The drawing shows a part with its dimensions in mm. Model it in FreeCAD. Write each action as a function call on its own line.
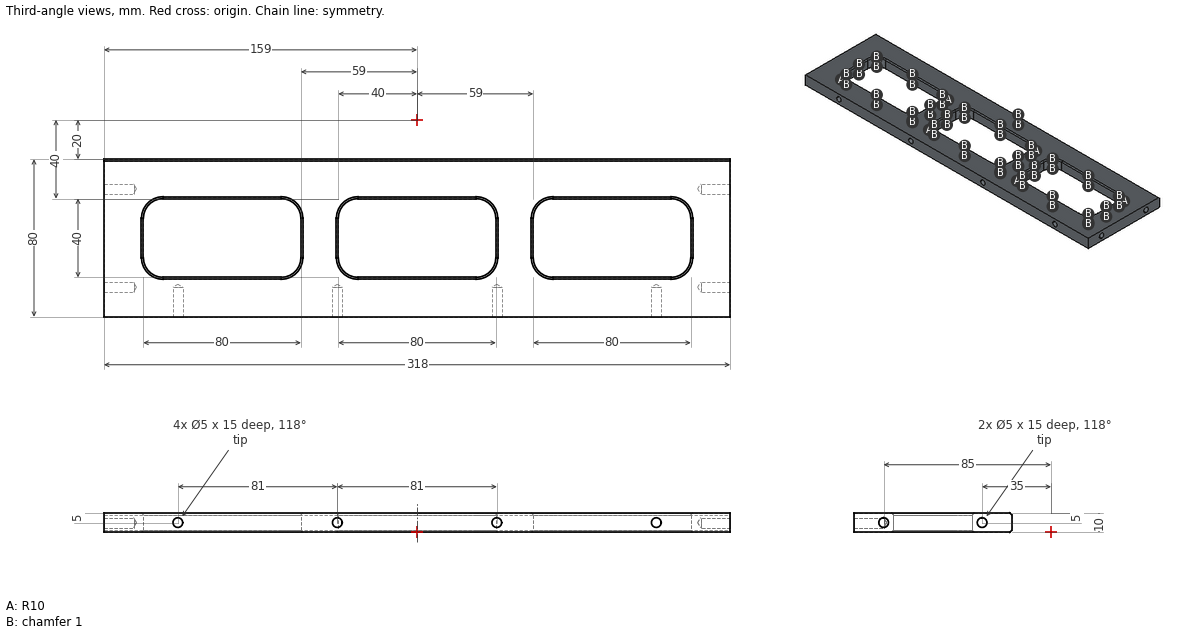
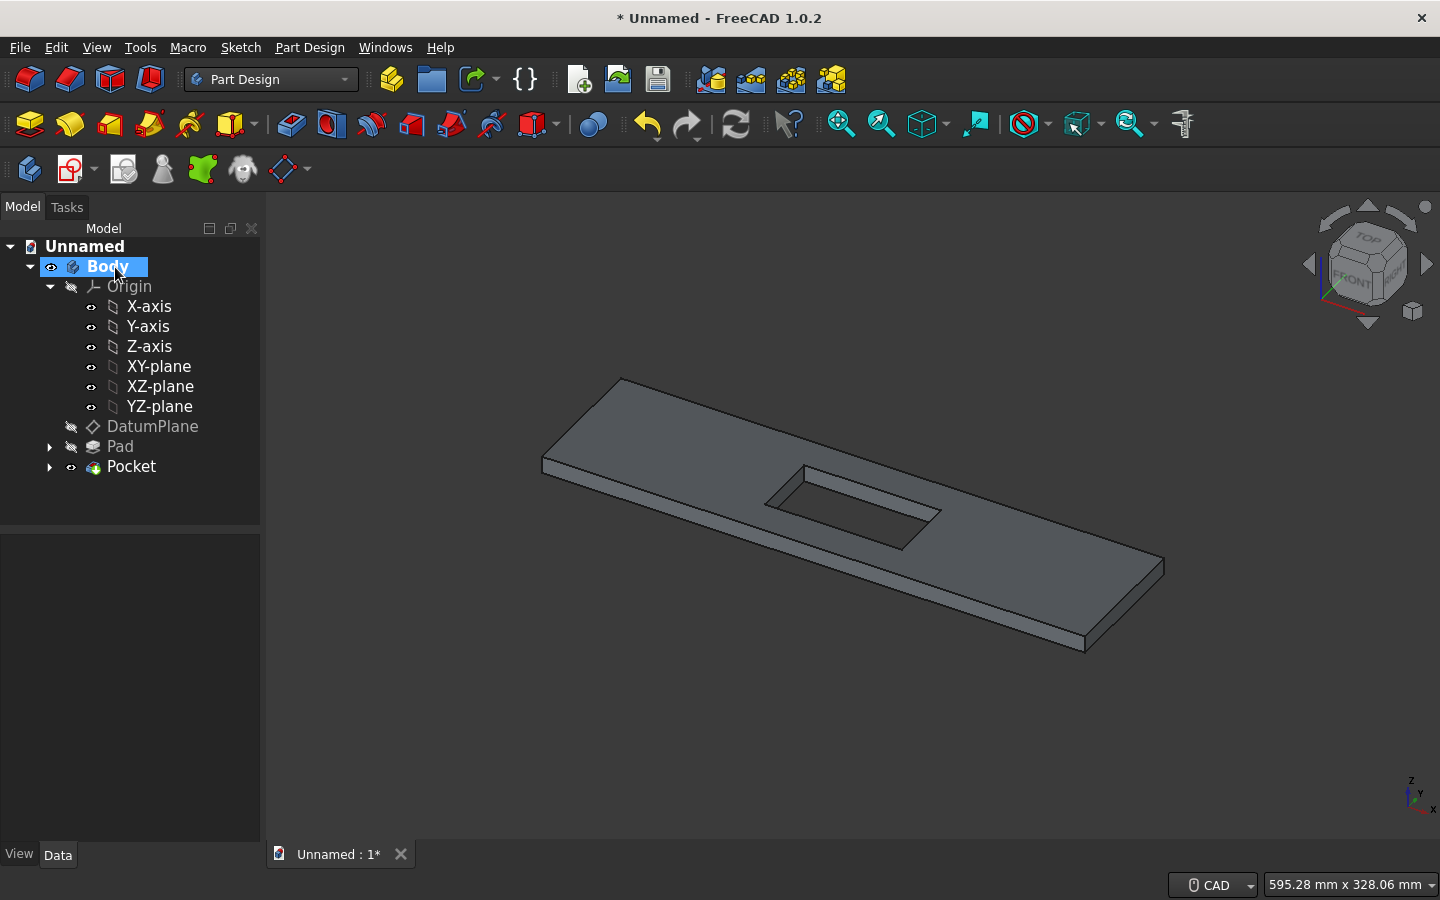
click(1008, 558)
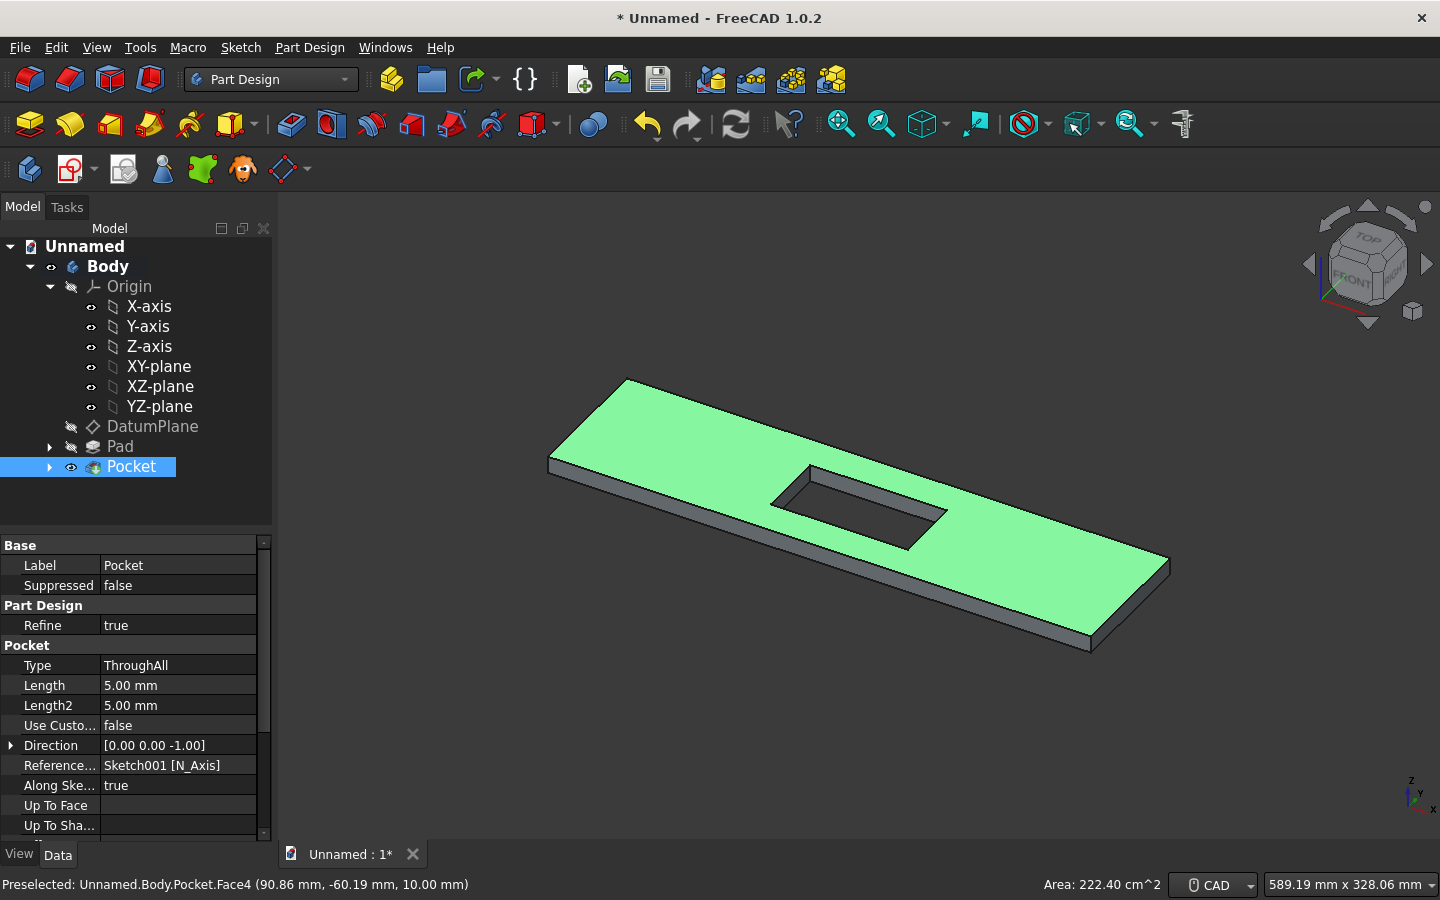
click(70, 170)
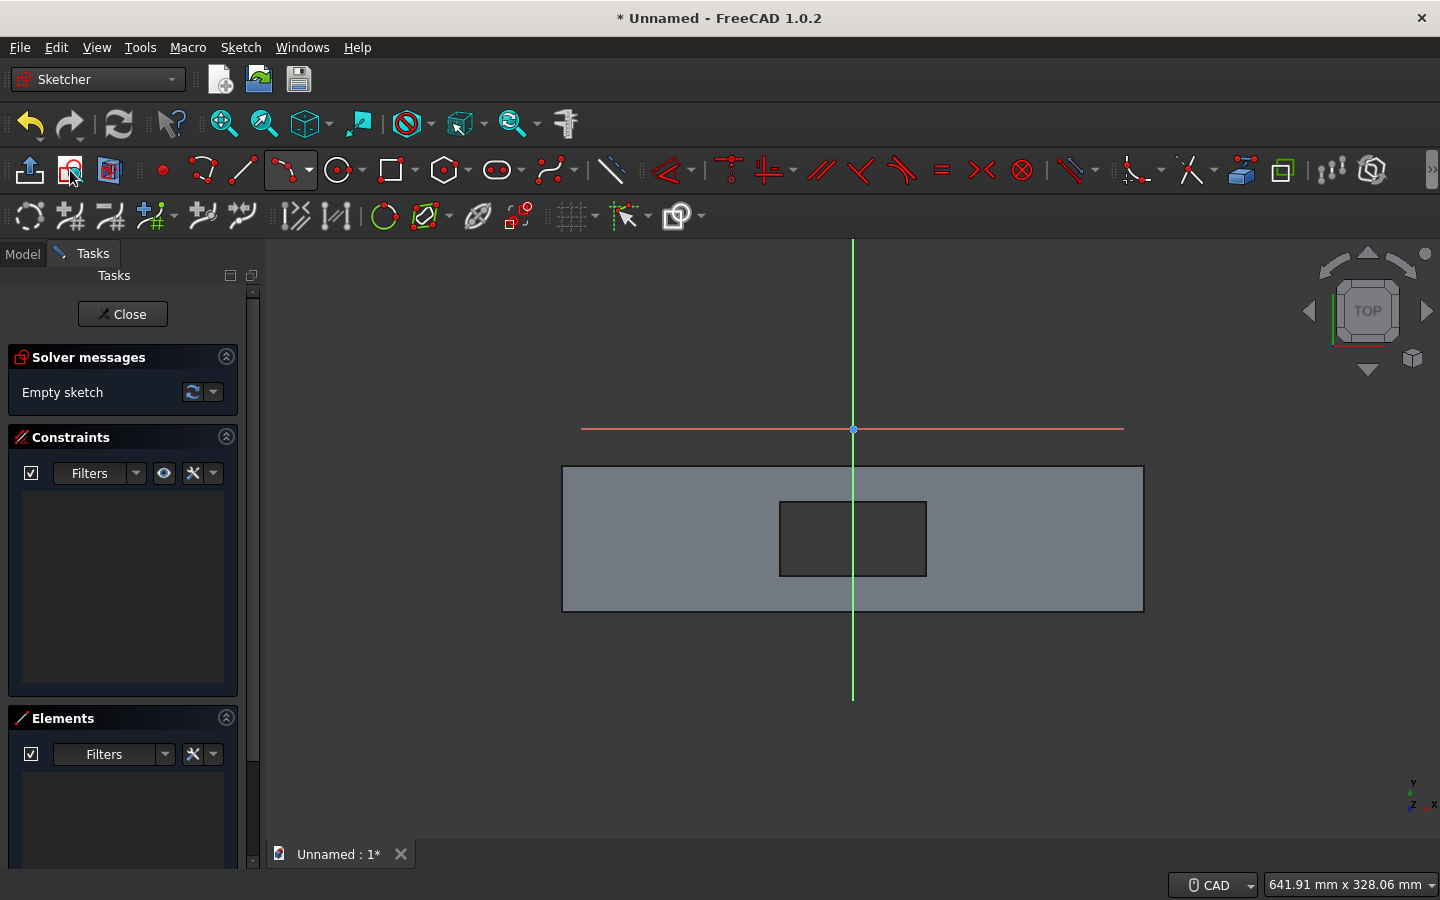
scroll(1094, 481, up, 5)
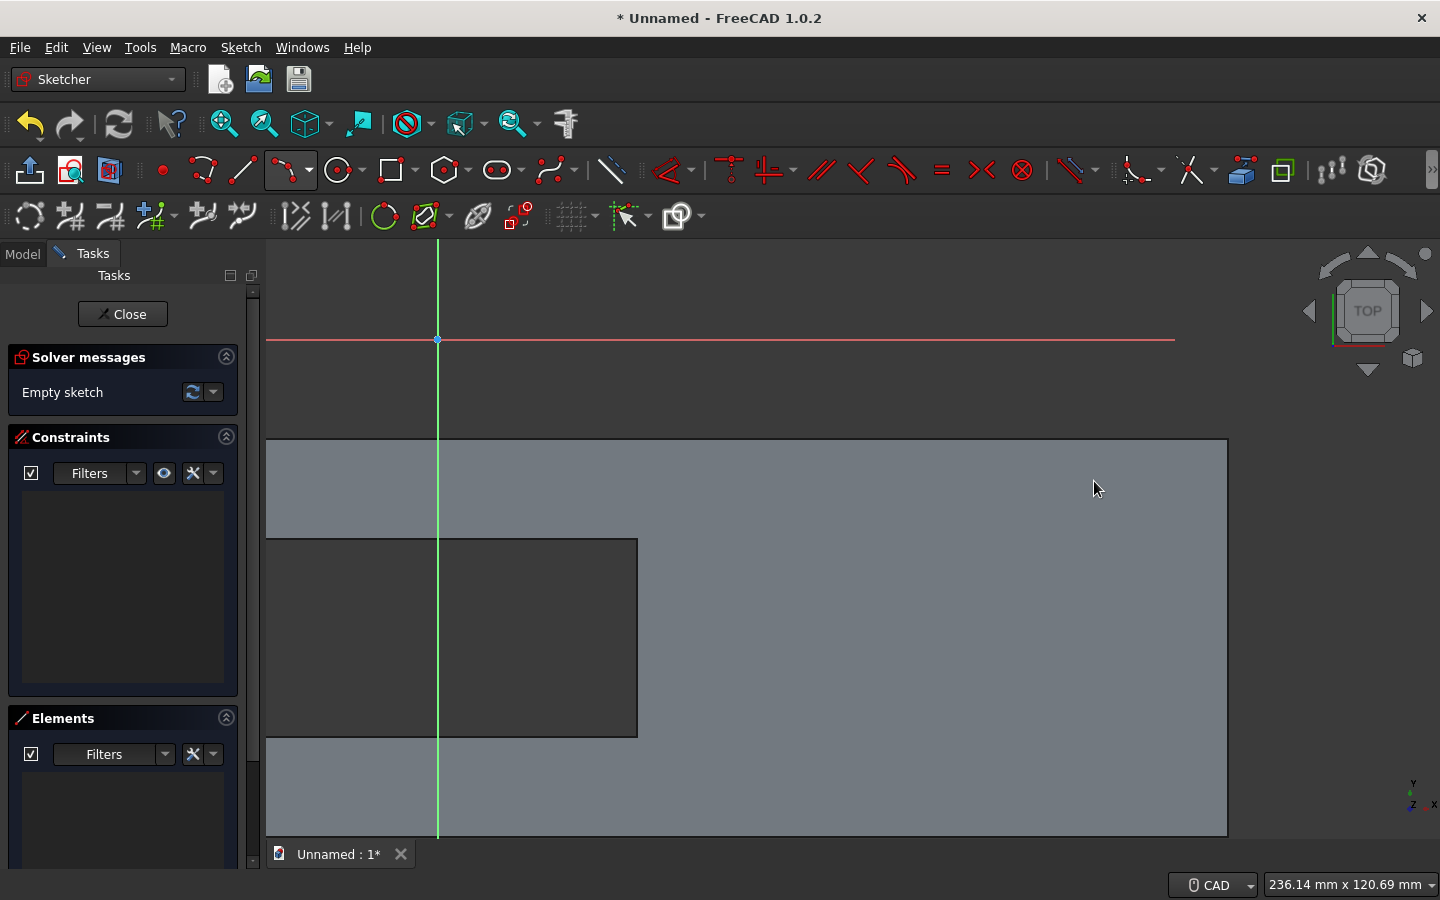
click(392, 170)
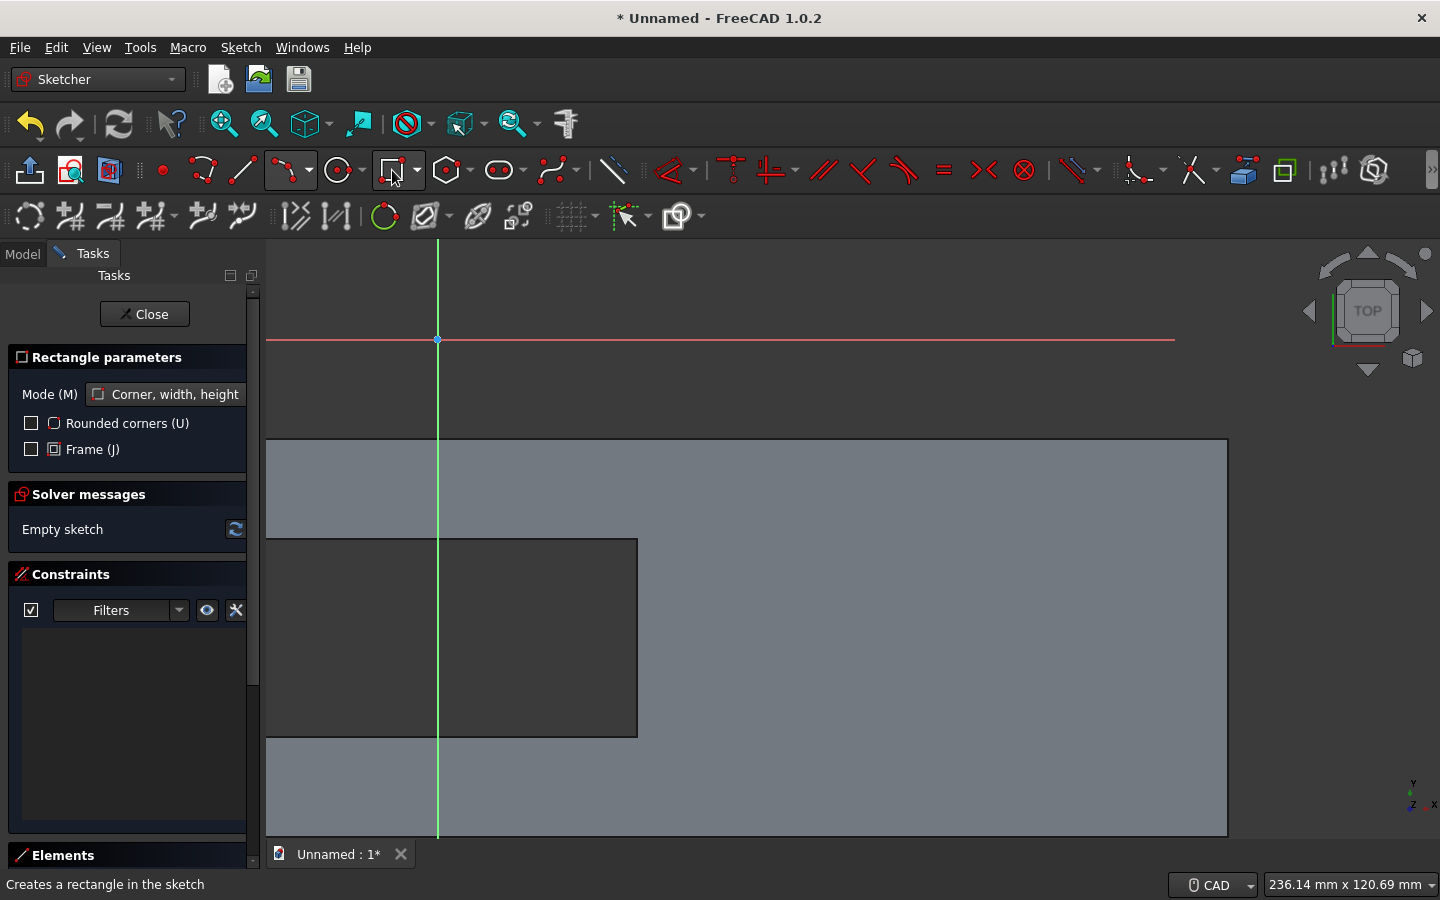
click(731, 539)
click(1129, 737)
key(Escape)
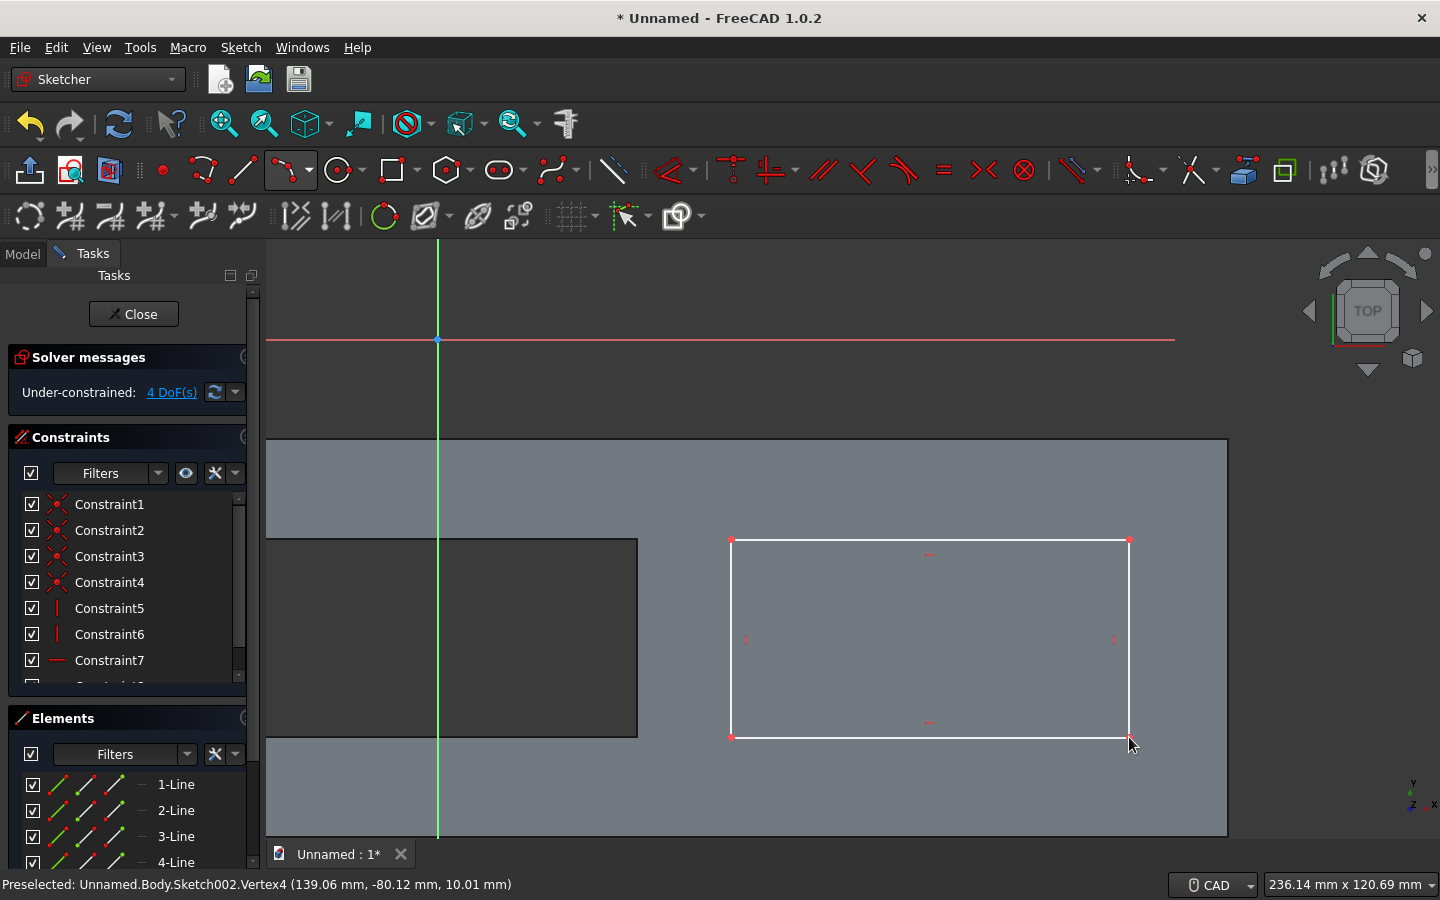
click(668, 170)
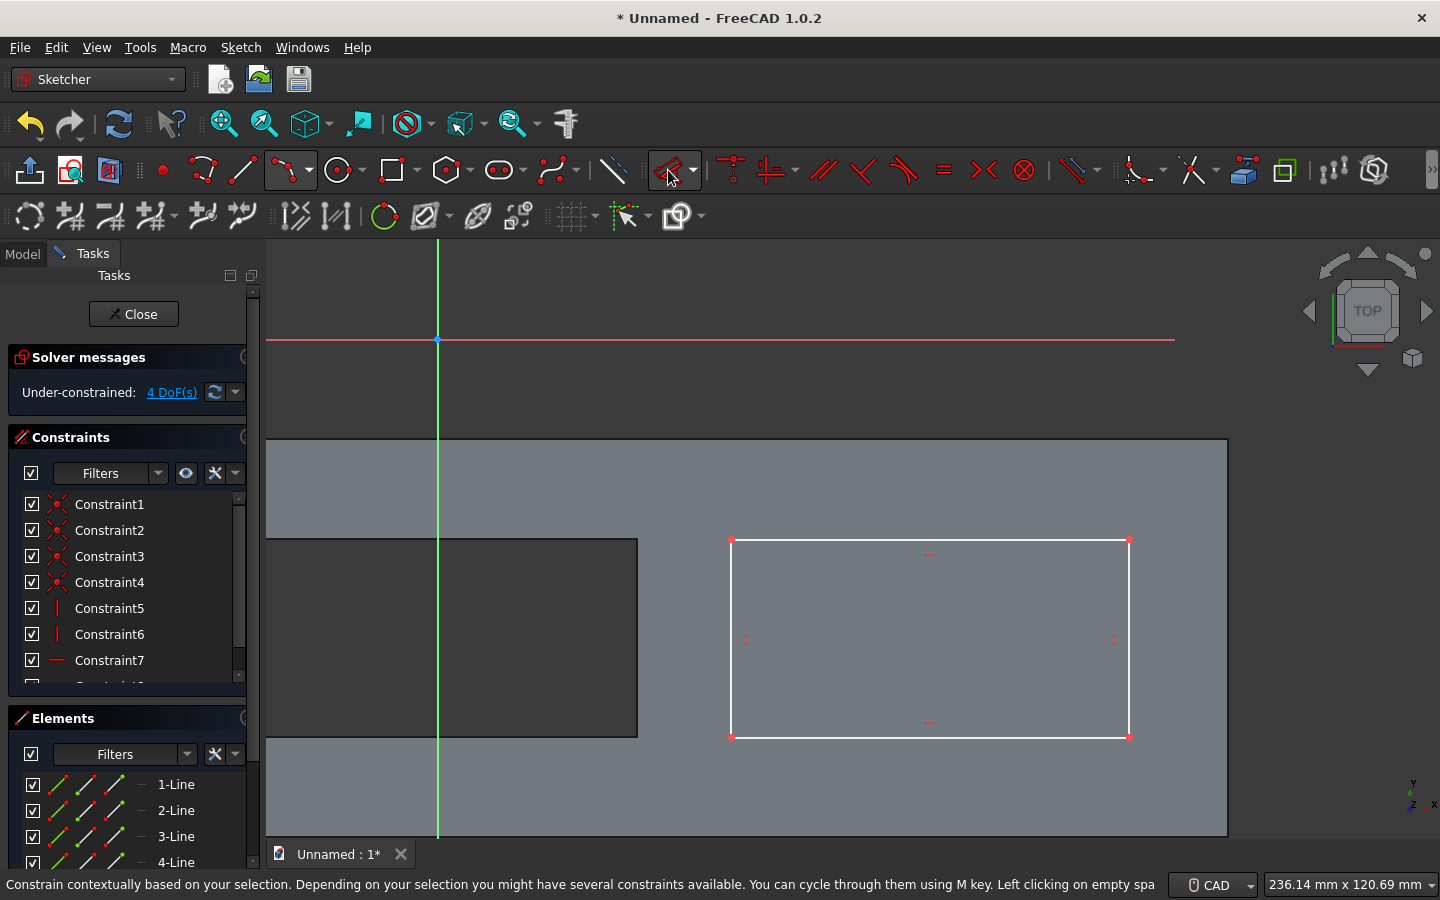
click(731, 599)
click(697, 639)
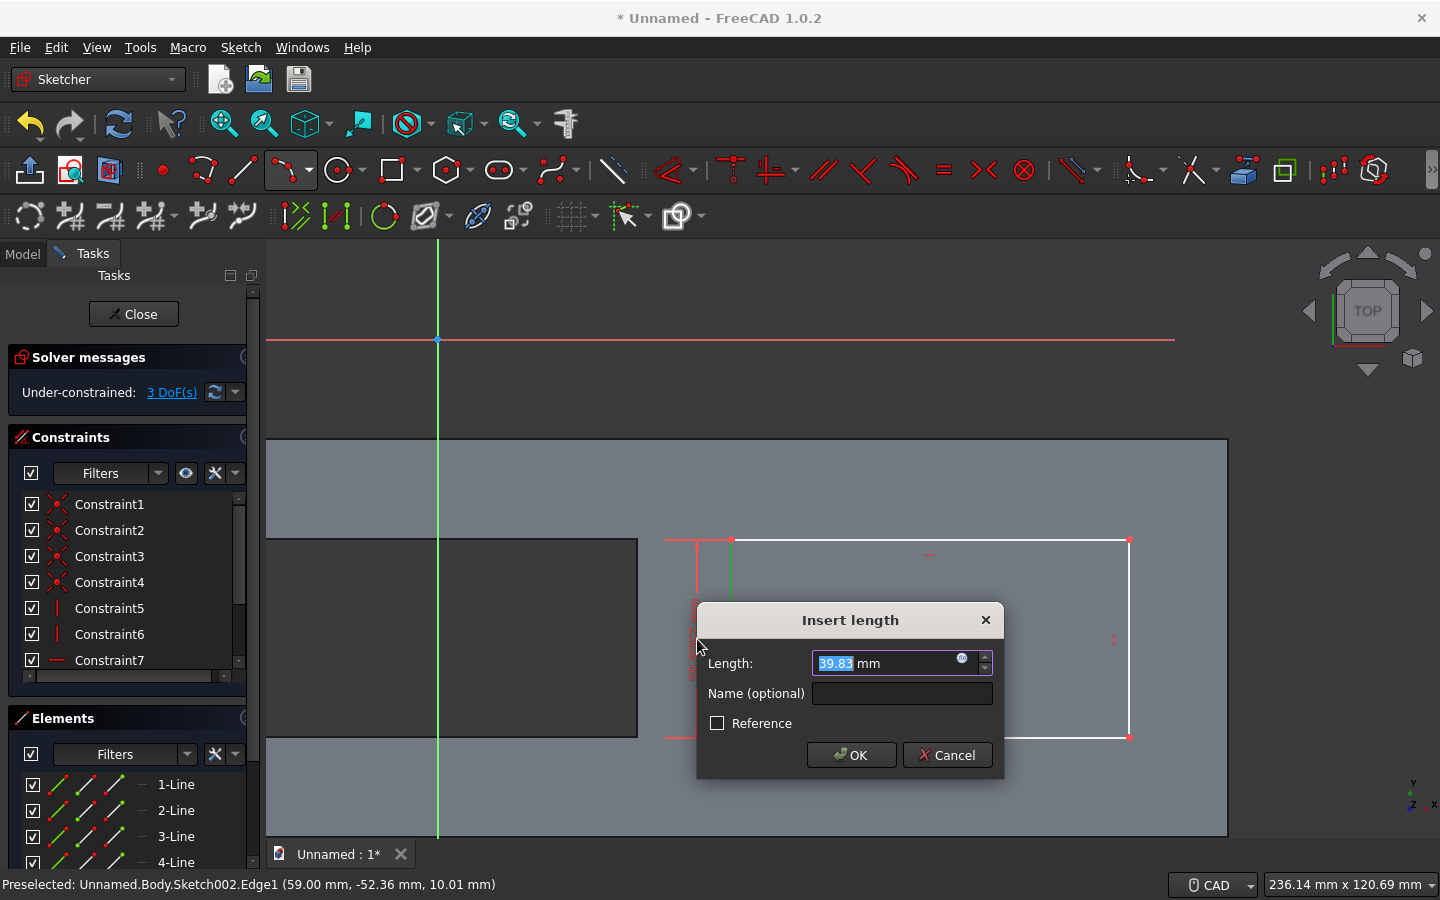
text(40)
key(Return)